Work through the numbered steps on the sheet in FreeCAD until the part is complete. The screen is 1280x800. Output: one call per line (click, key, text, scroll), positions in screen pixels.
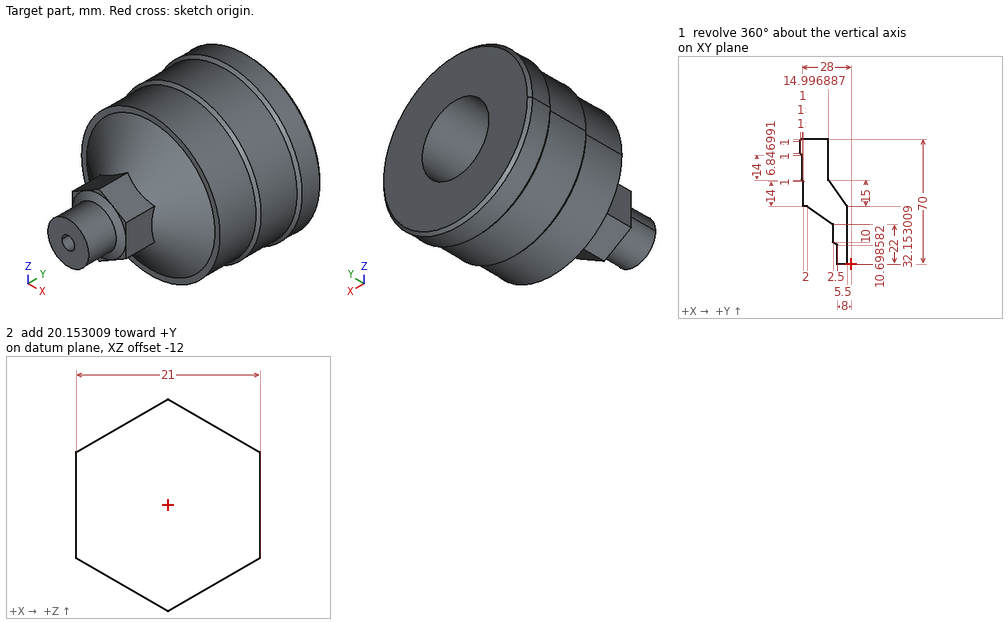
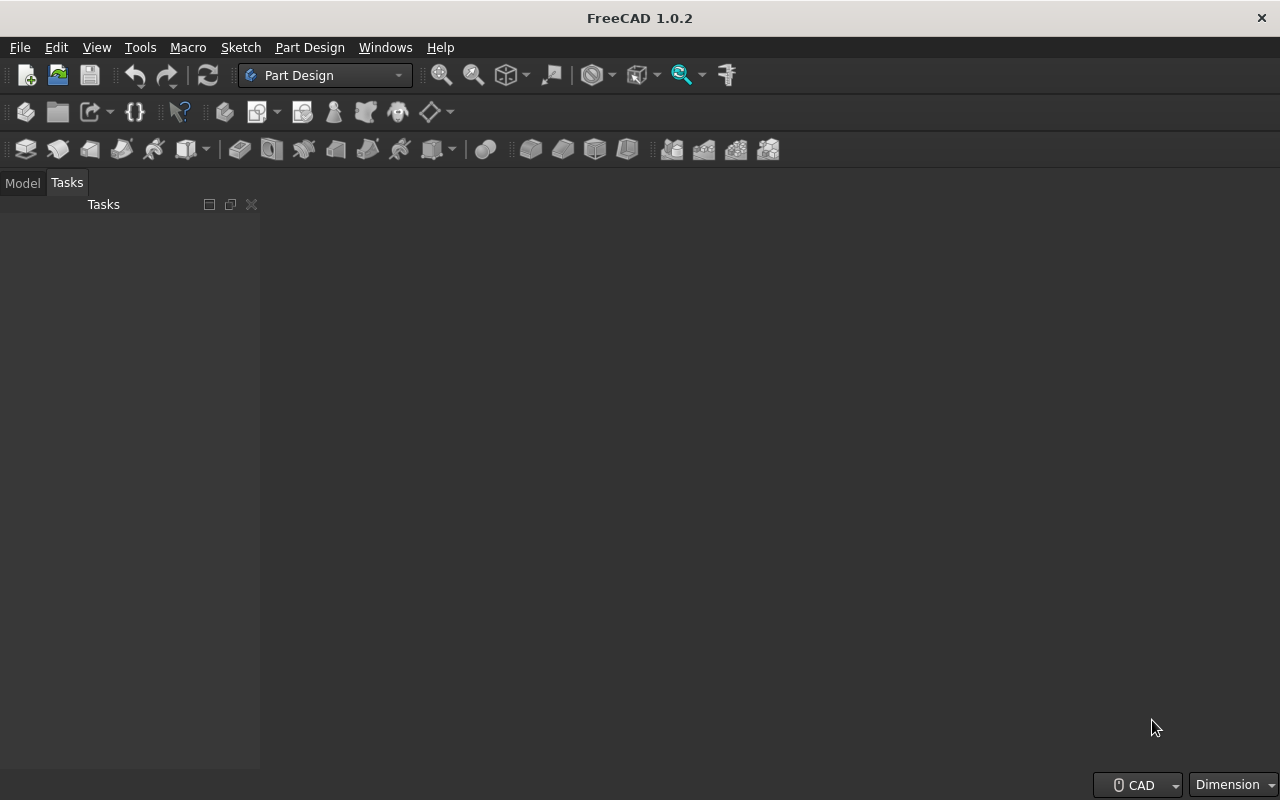
click(26, 76)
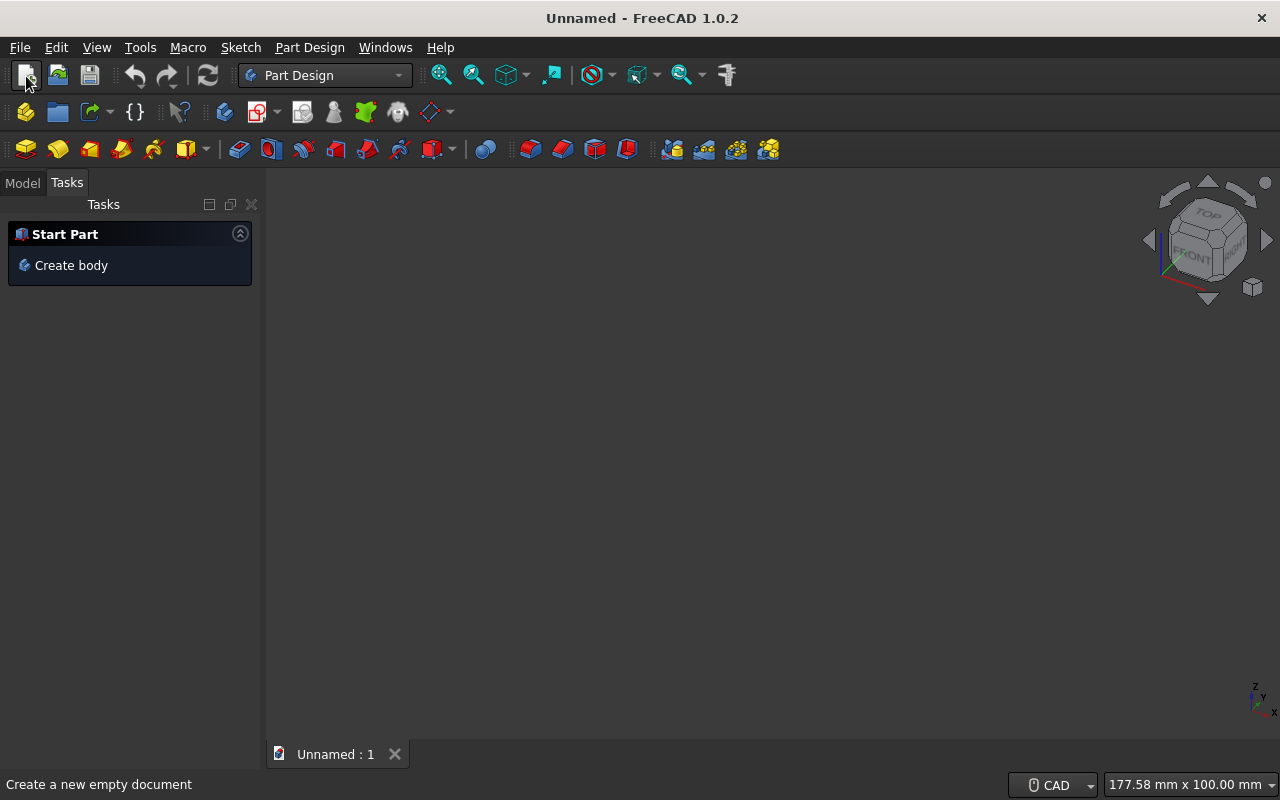
click(258, 112)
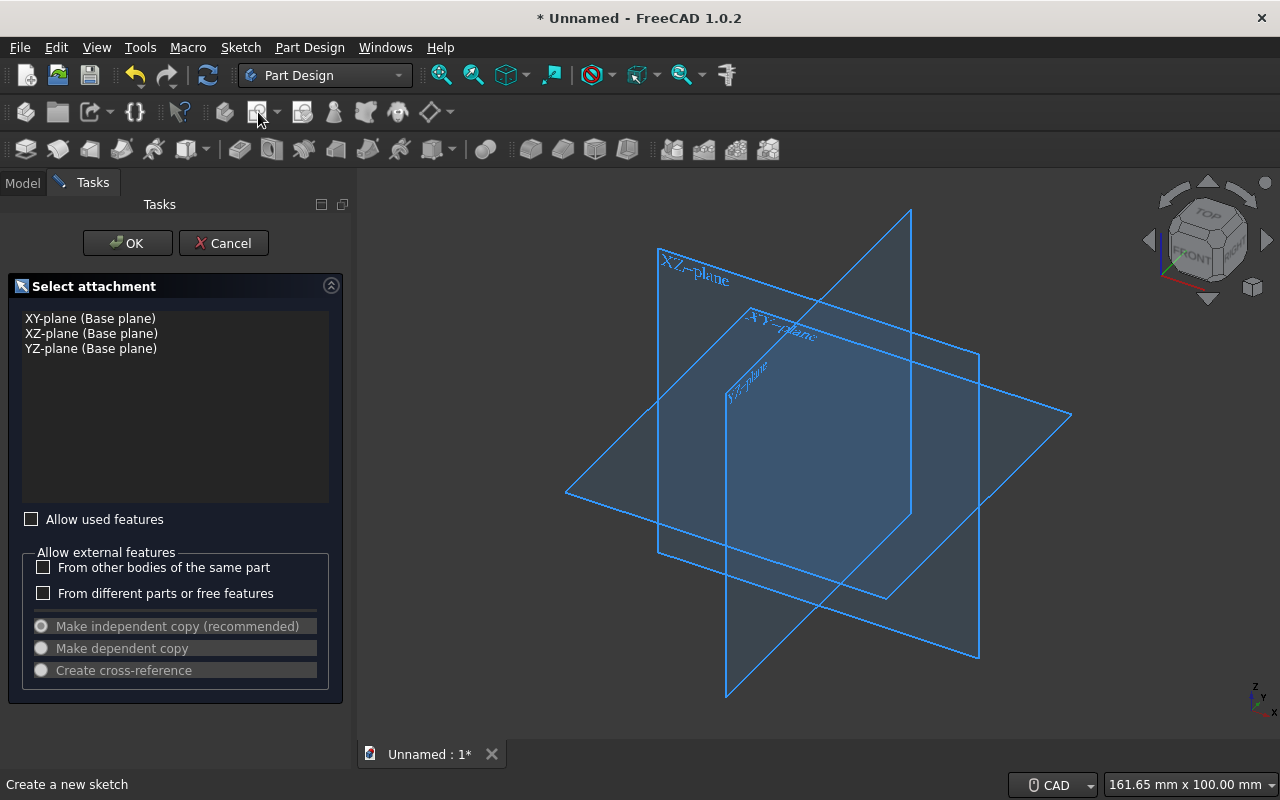
click(82, 318)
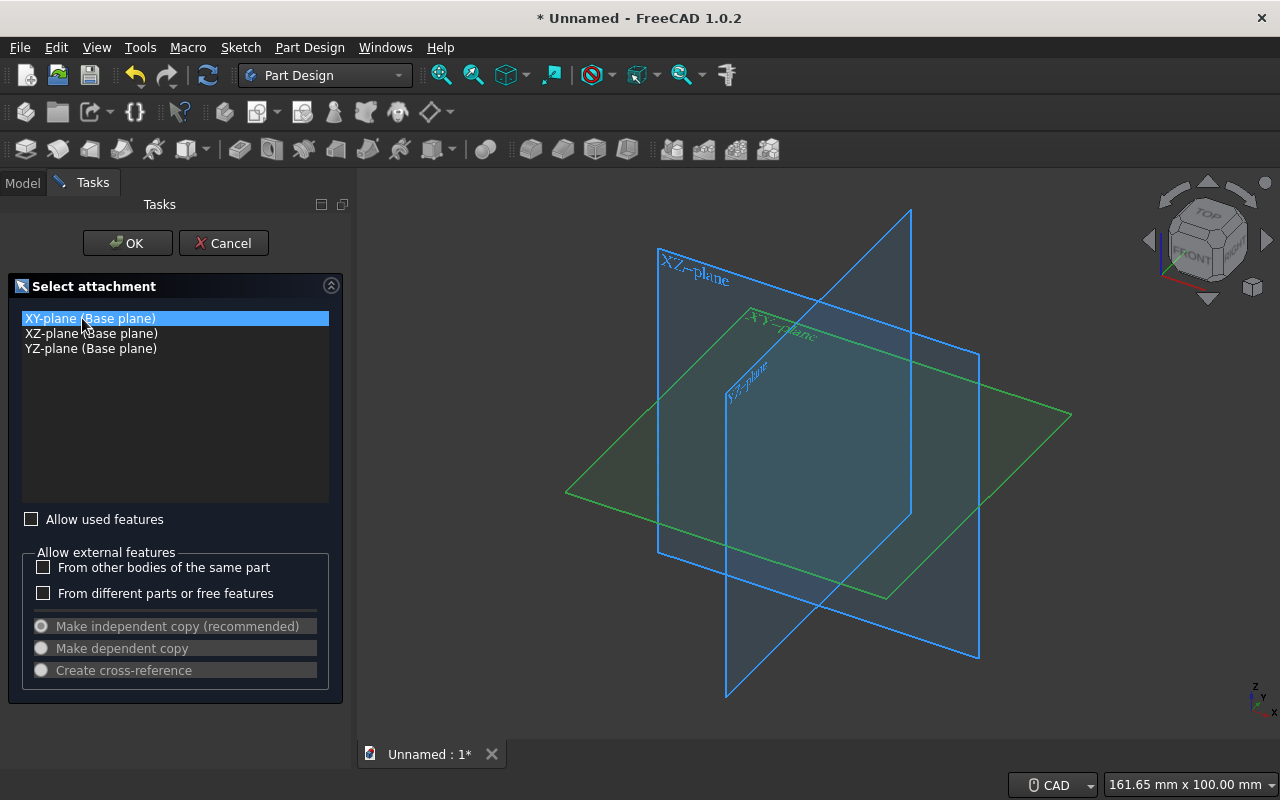
click(128, 243)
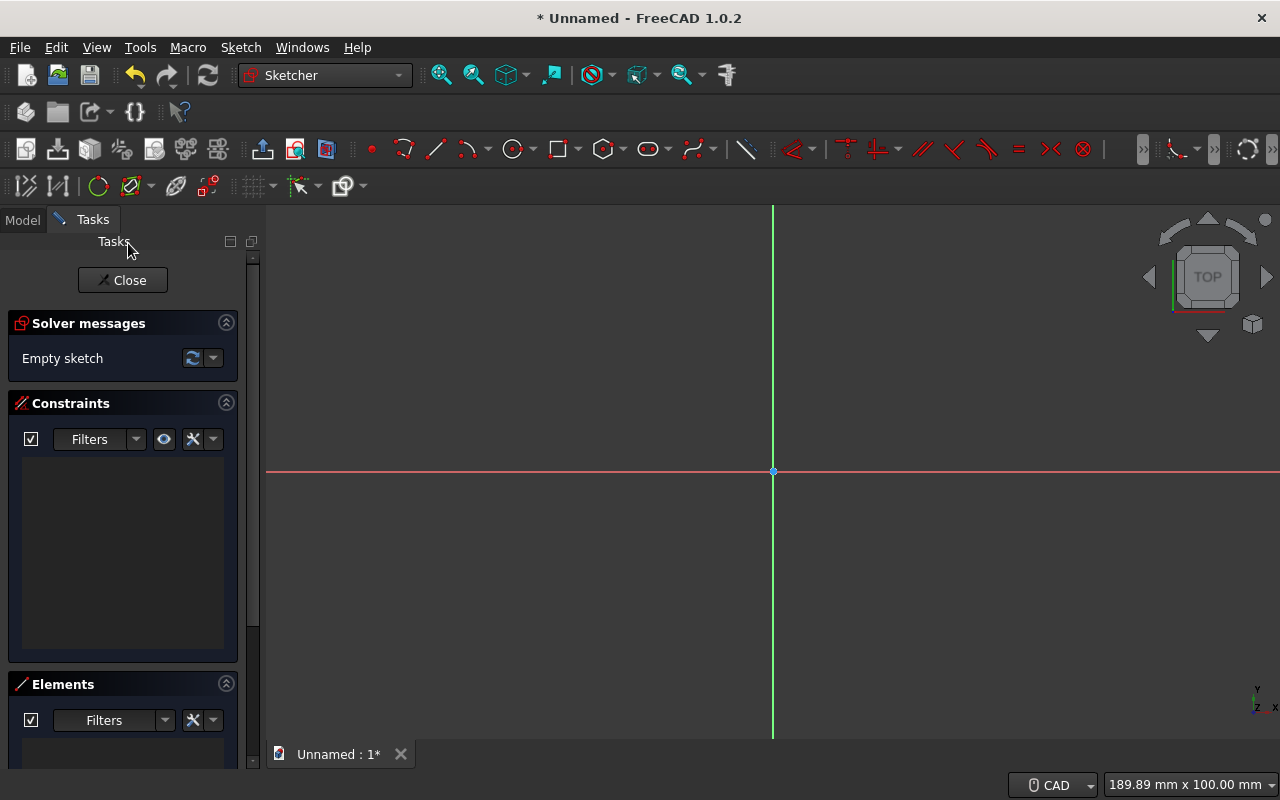
scroll(723, 711, down, 2)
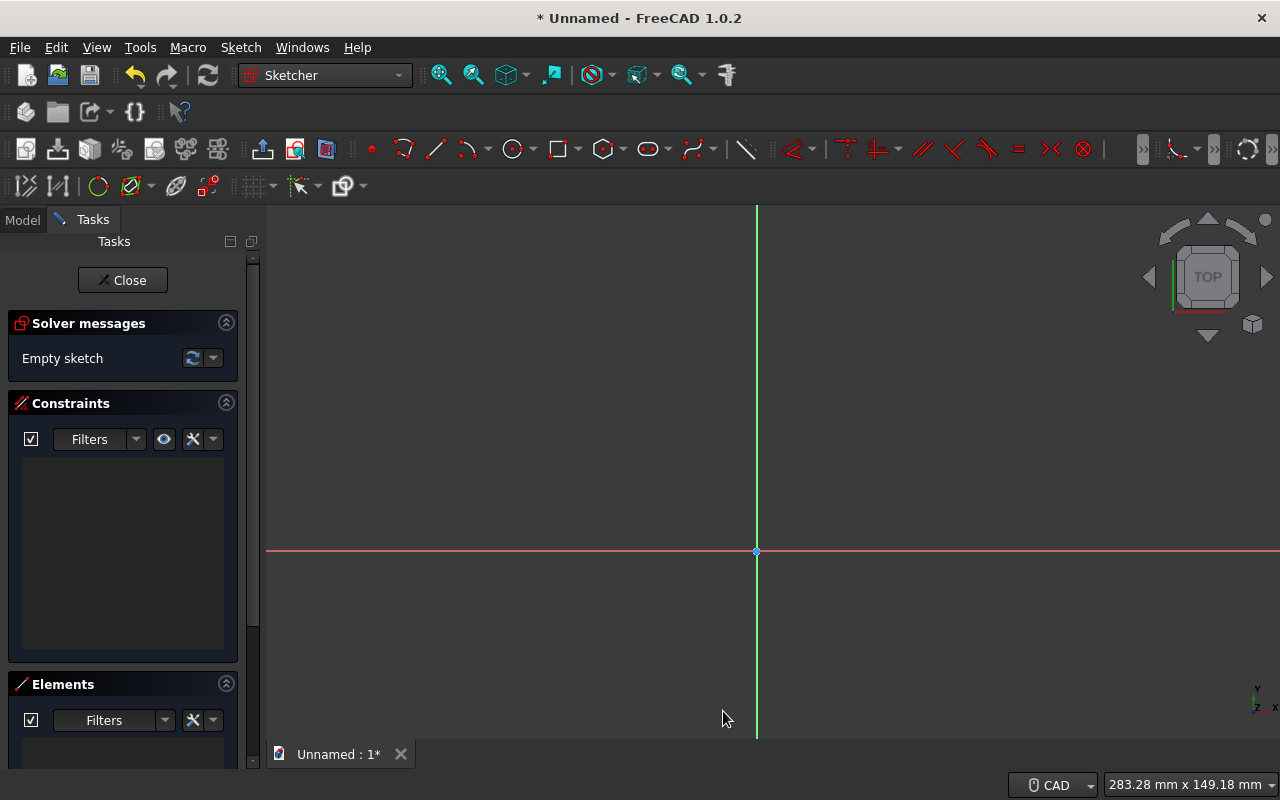
key(g)
key(m)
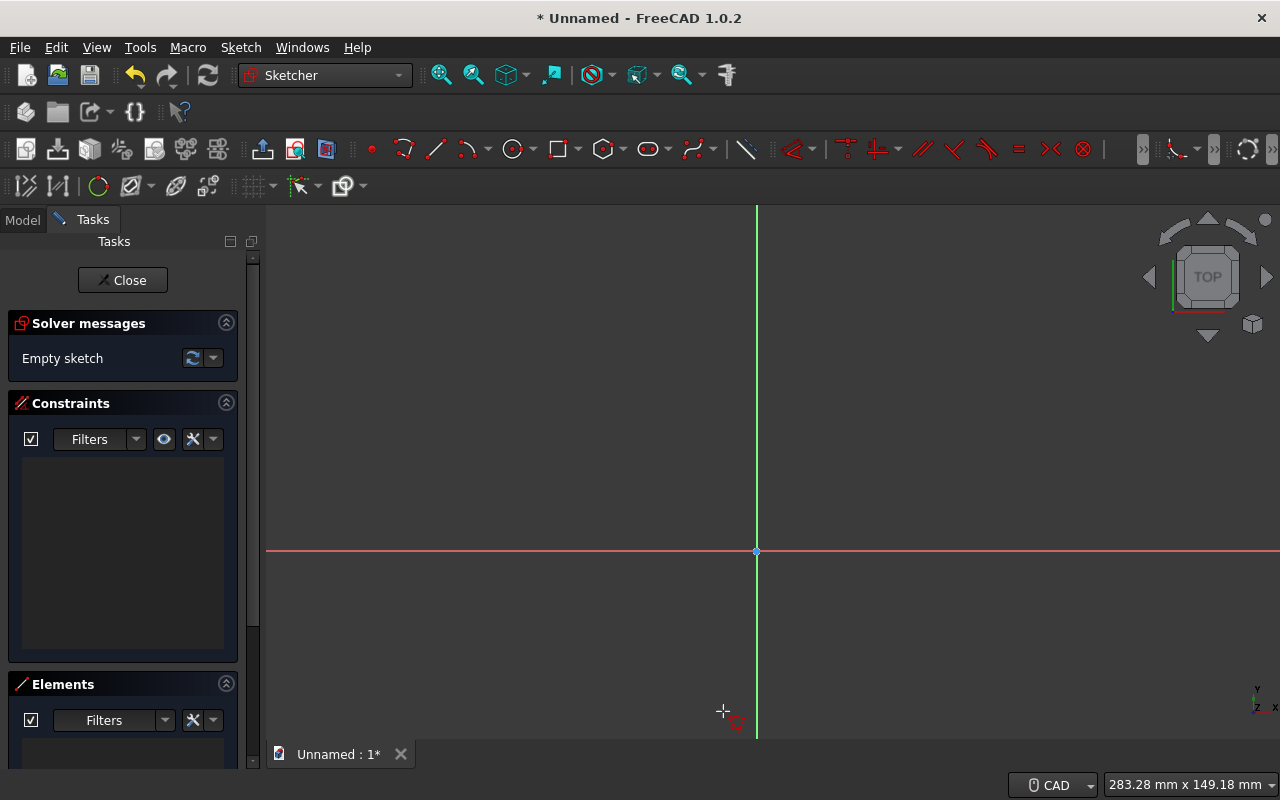
scroll(748, 551, up, 3)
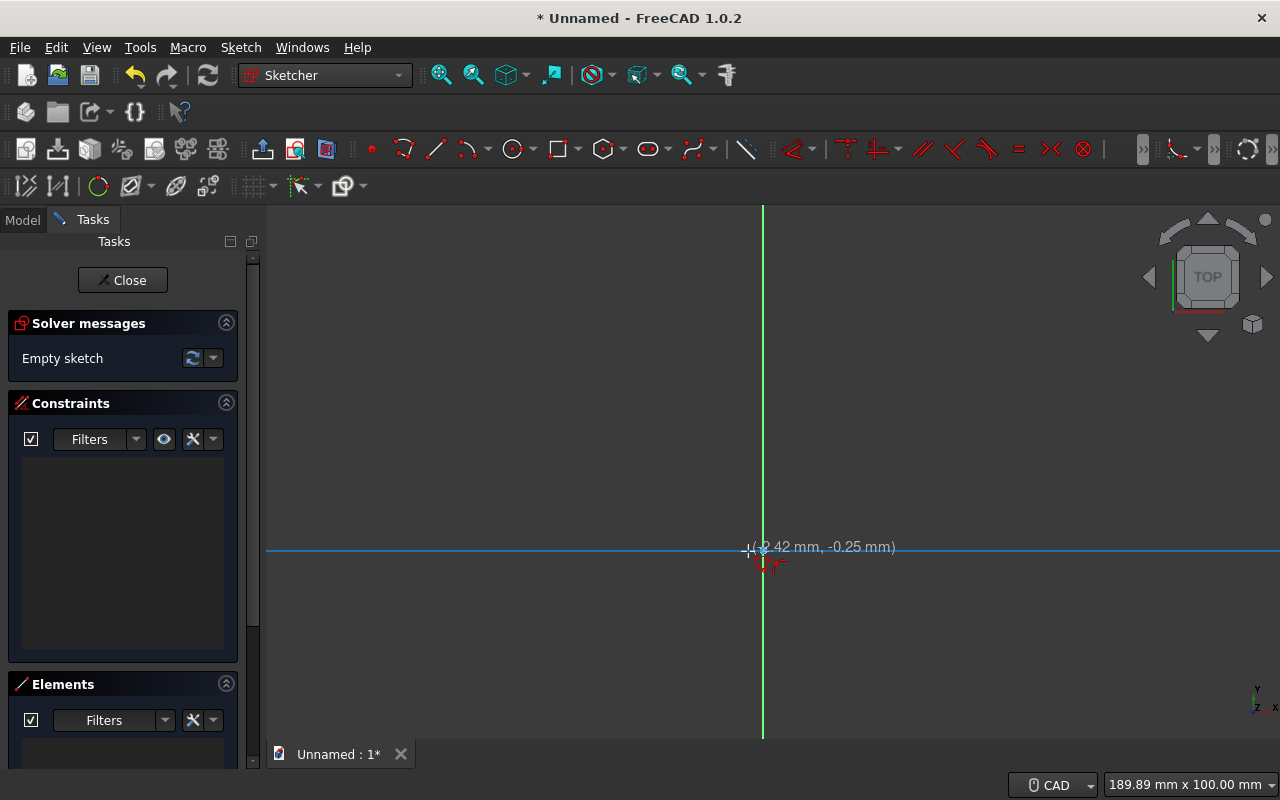
click(747, 551)
click(747, 341)
click(679, 243)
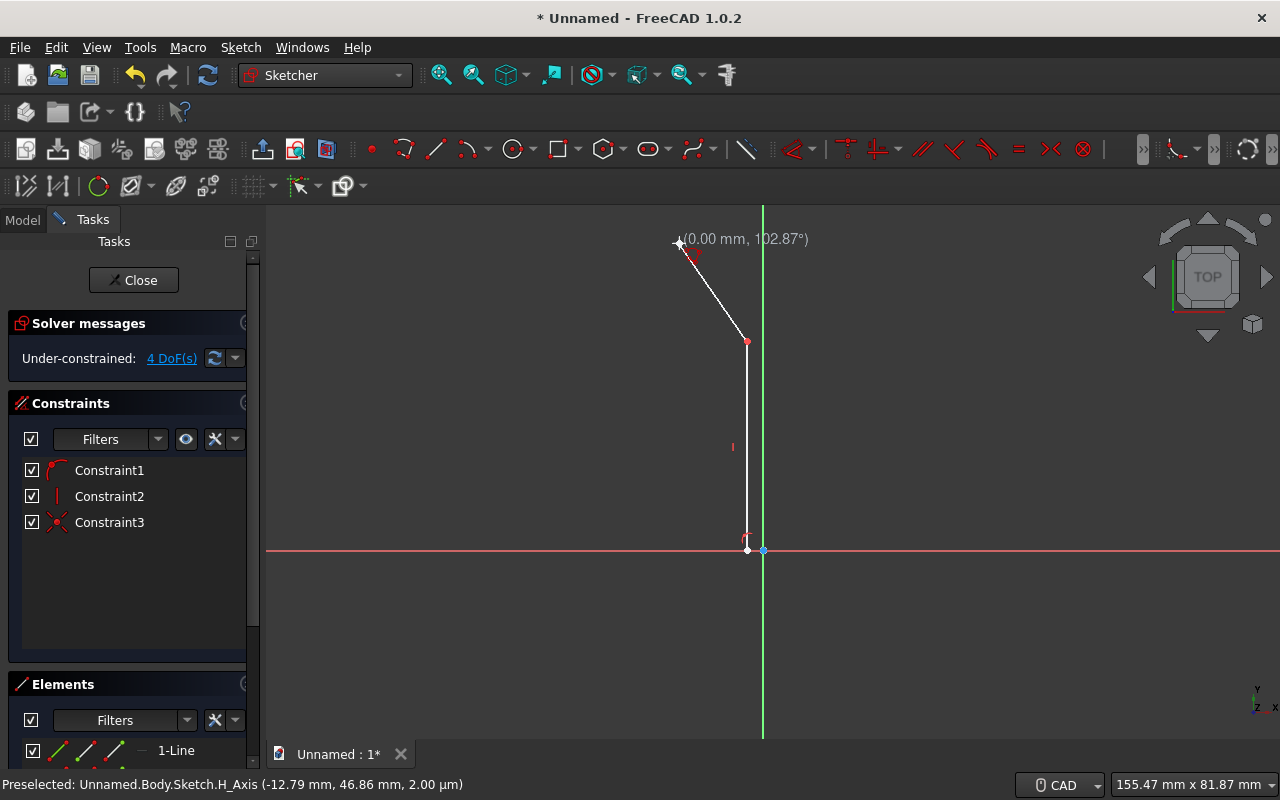
scroll(777, 711, down, 2)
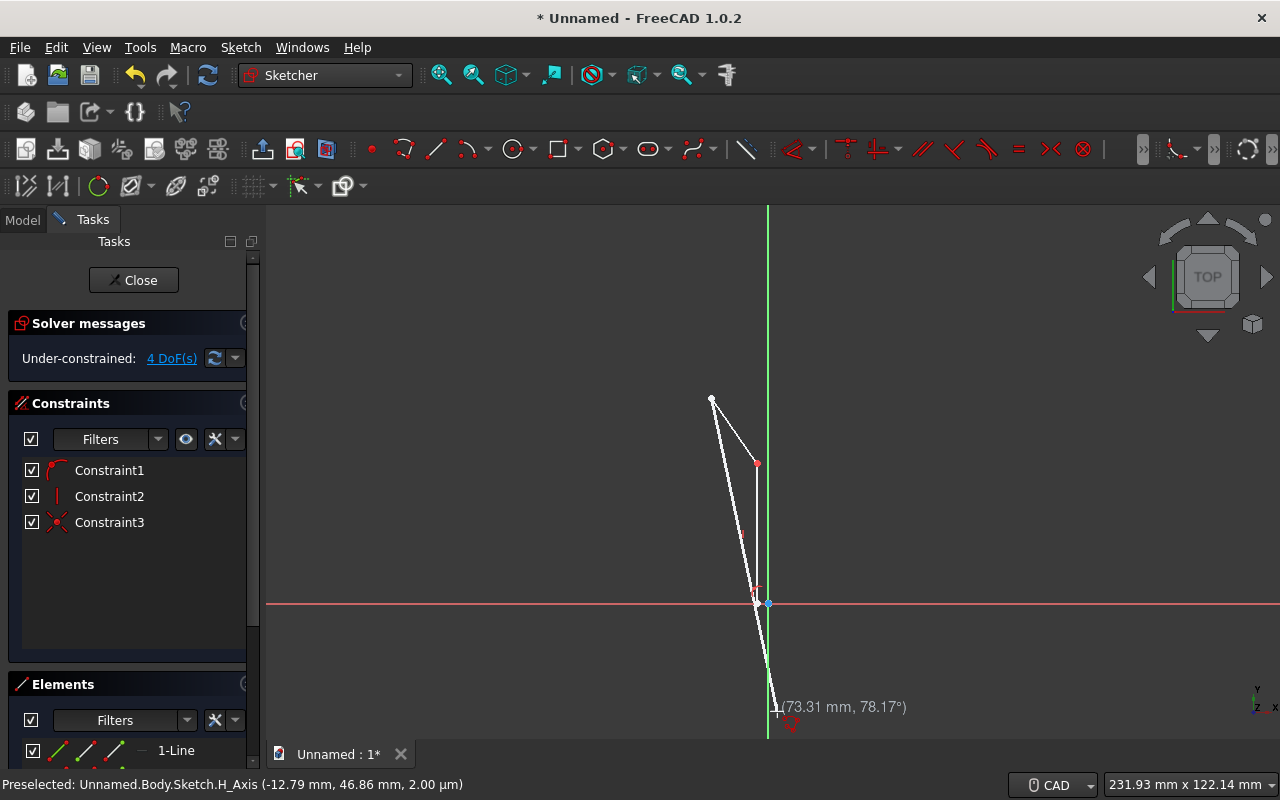
click(711, 298)
click(646, 298)